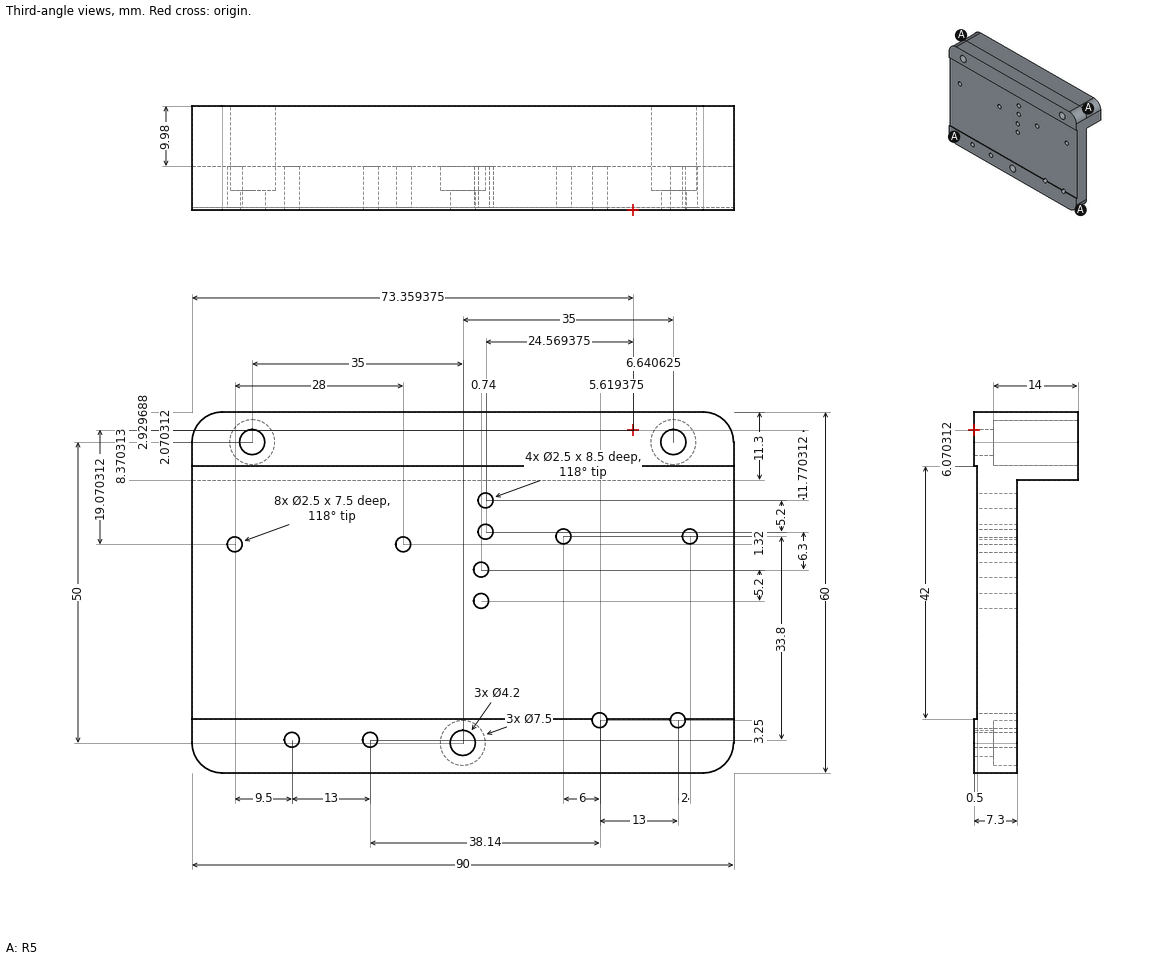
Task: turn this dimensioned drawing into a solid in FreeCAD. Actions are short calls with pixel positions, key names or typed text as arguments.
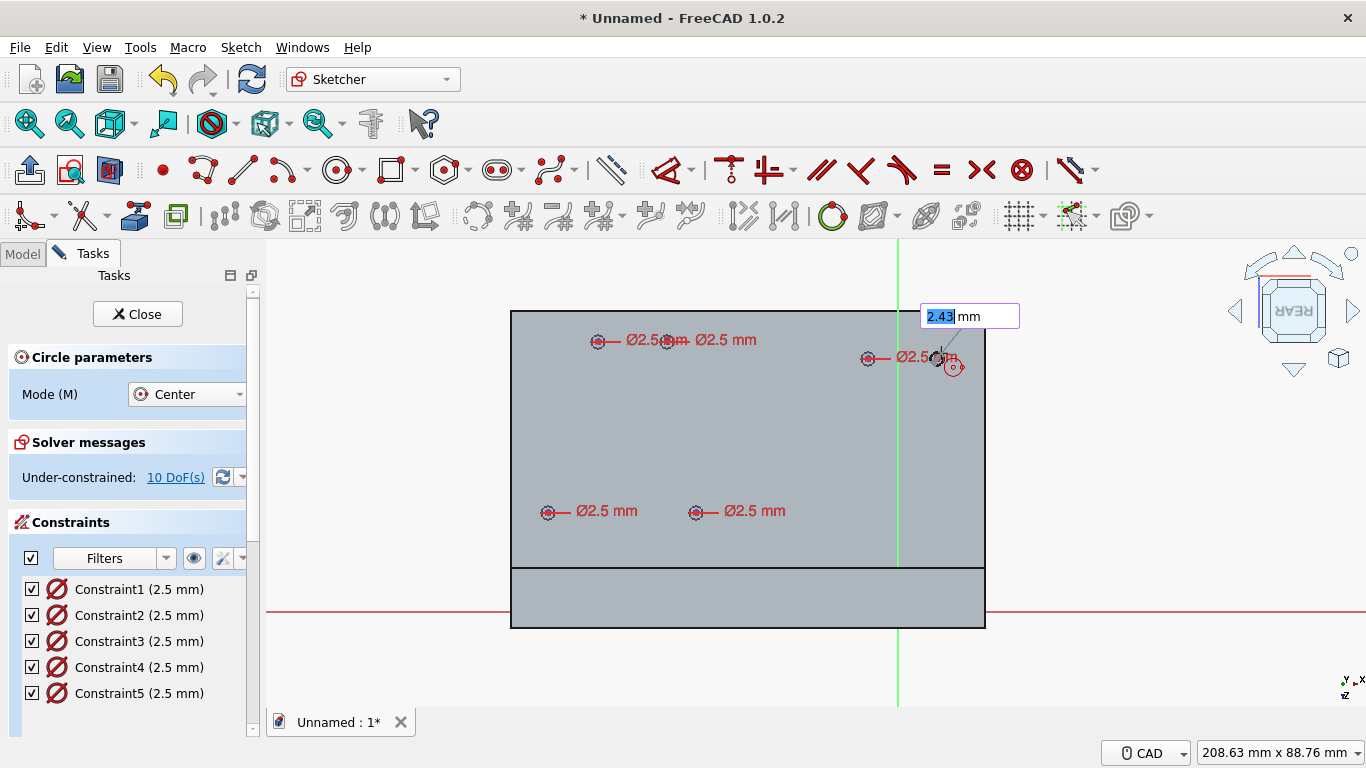
text(2.5)
key(Return)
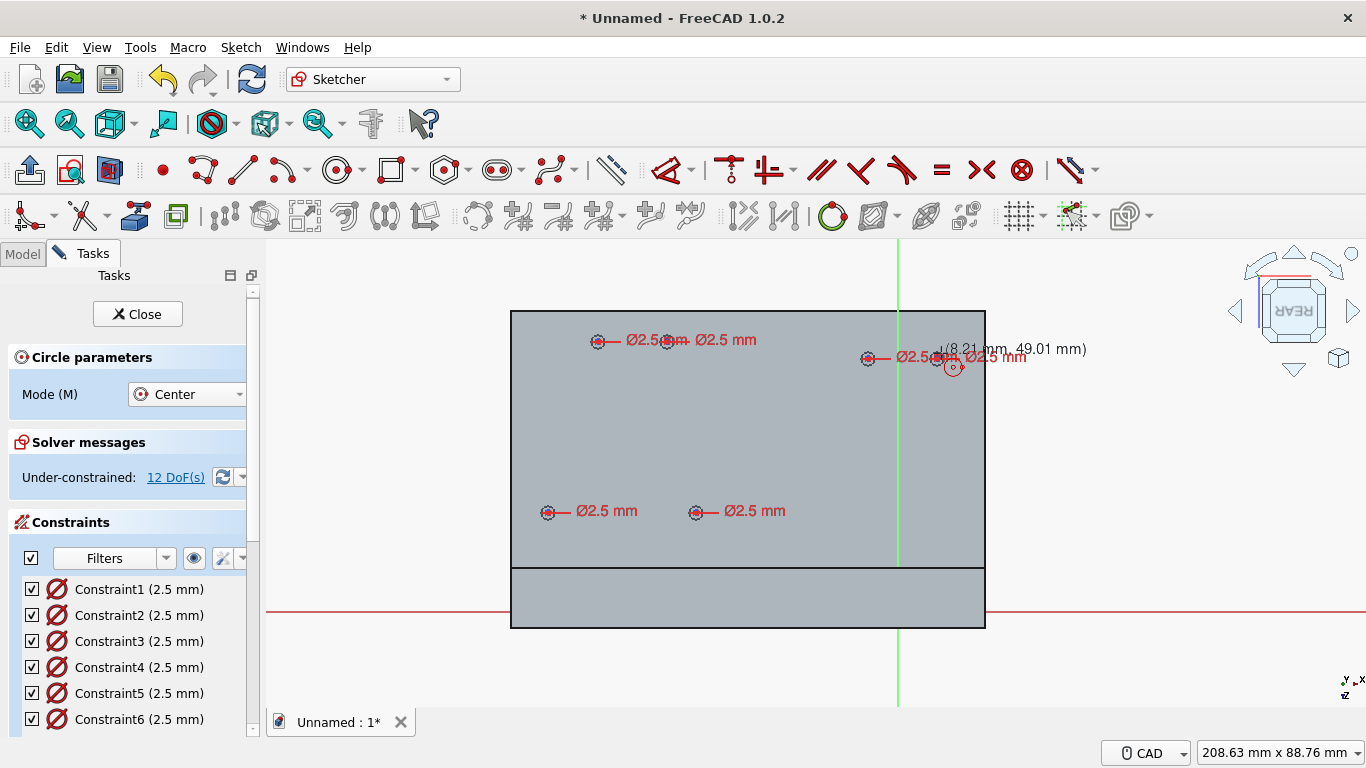
scroll(836, 519, up, 7)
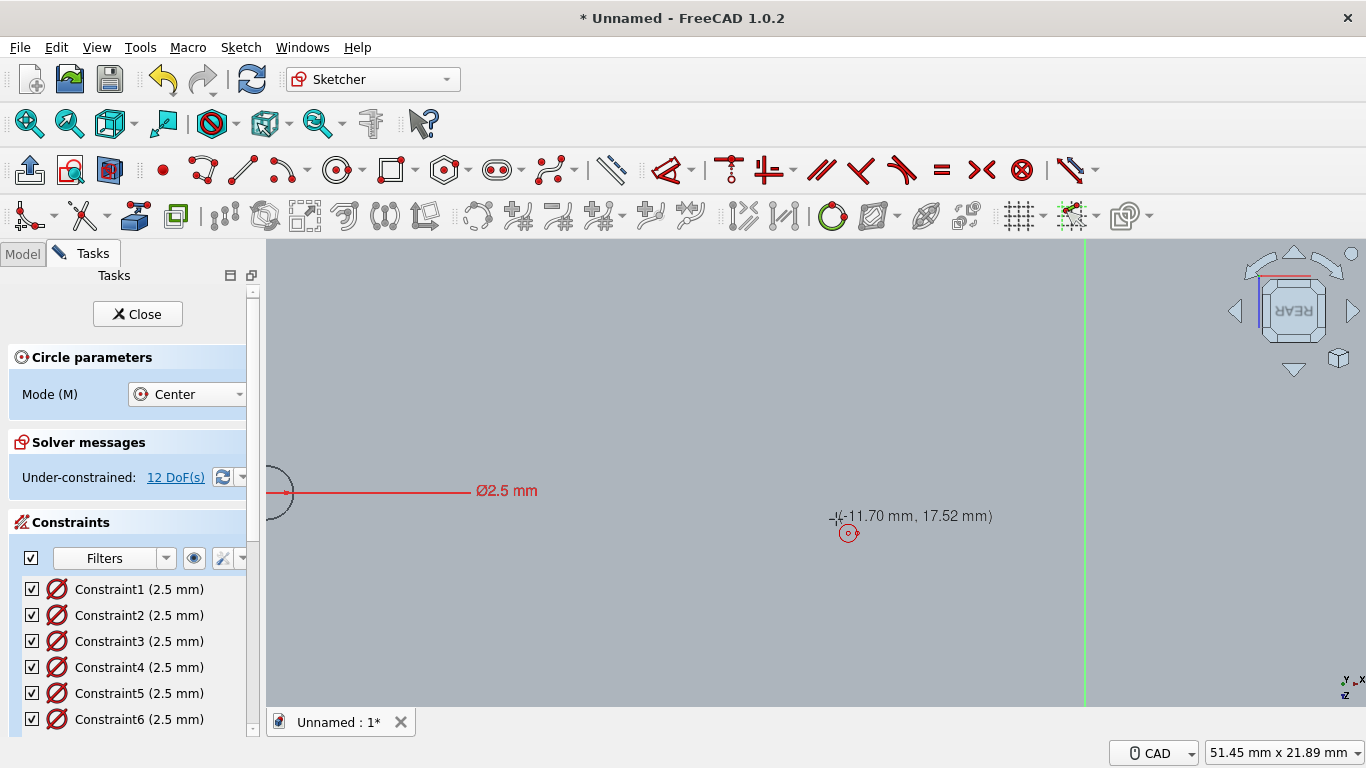
scroll(836, 519, down, 7)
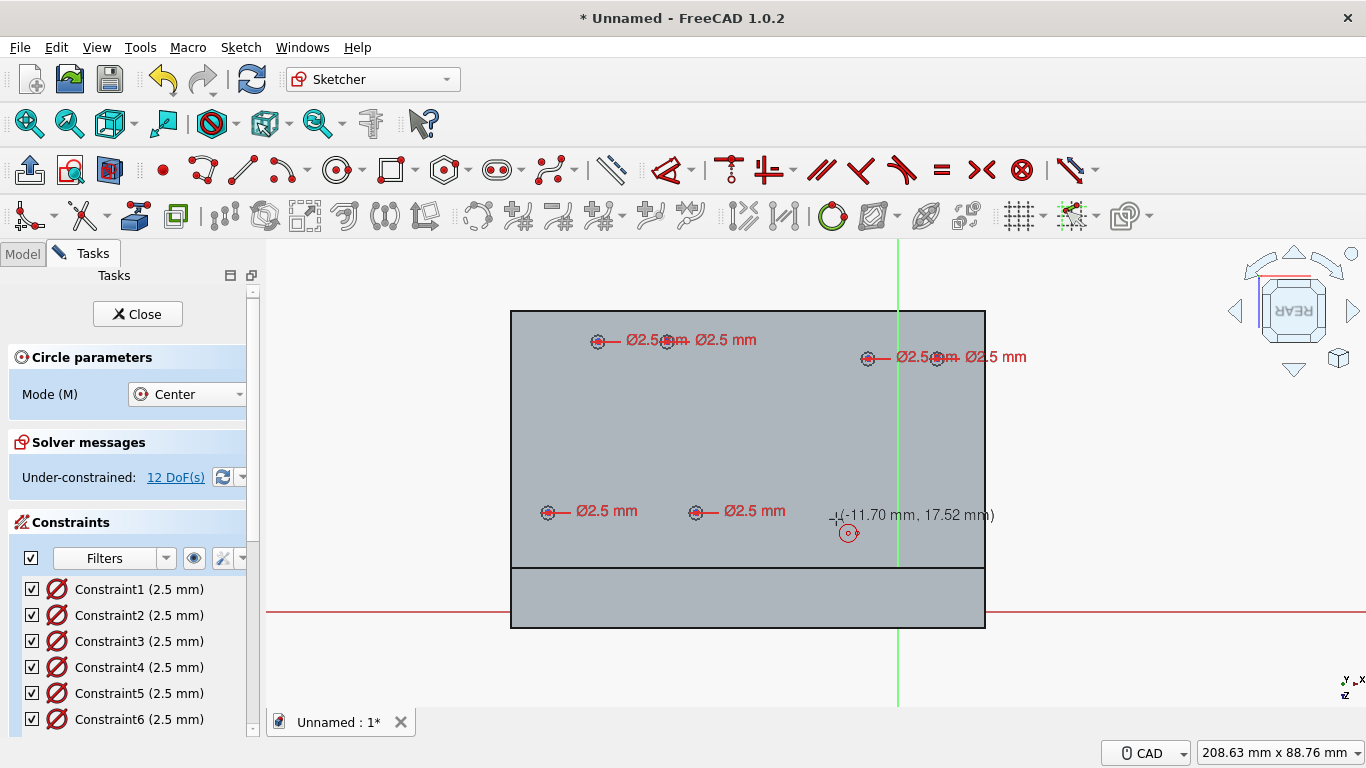
click(836, 519)
move(841, 514)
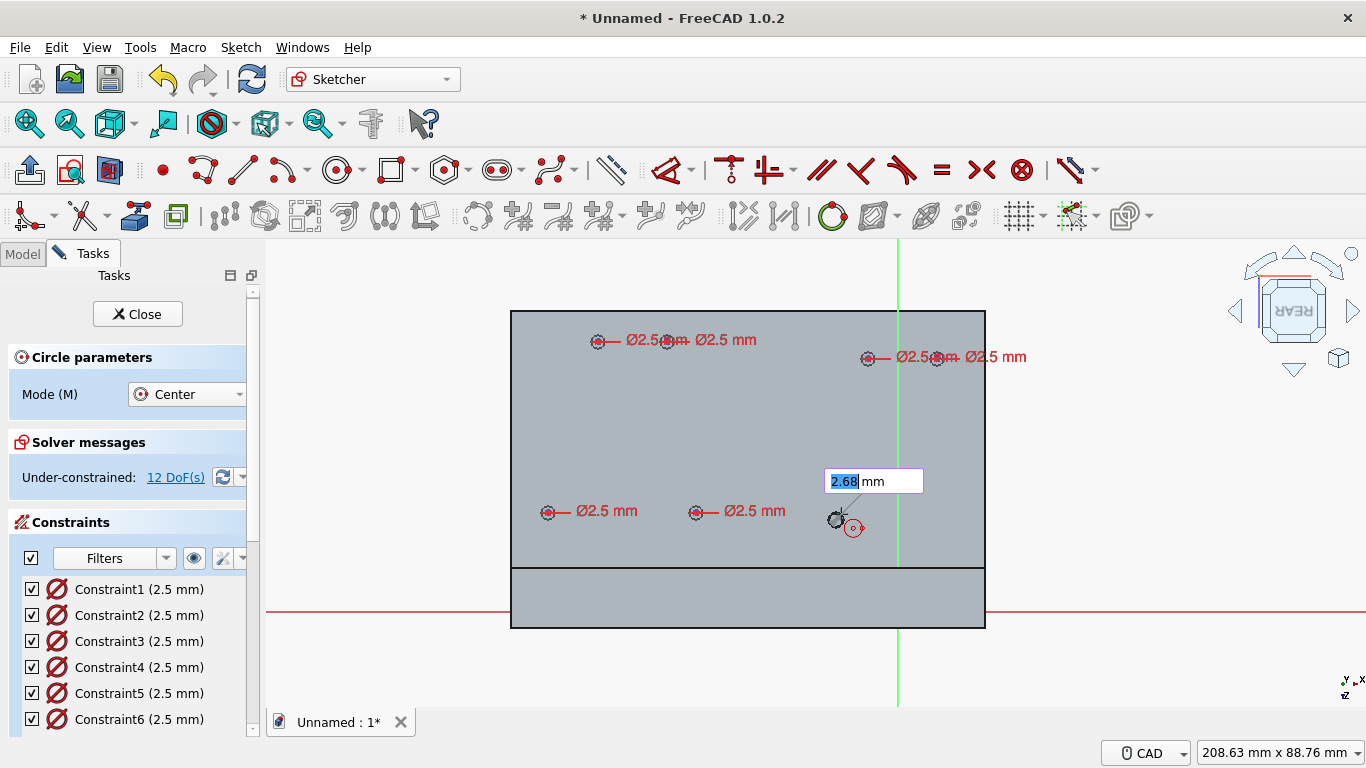
text(2.5)
key(Return)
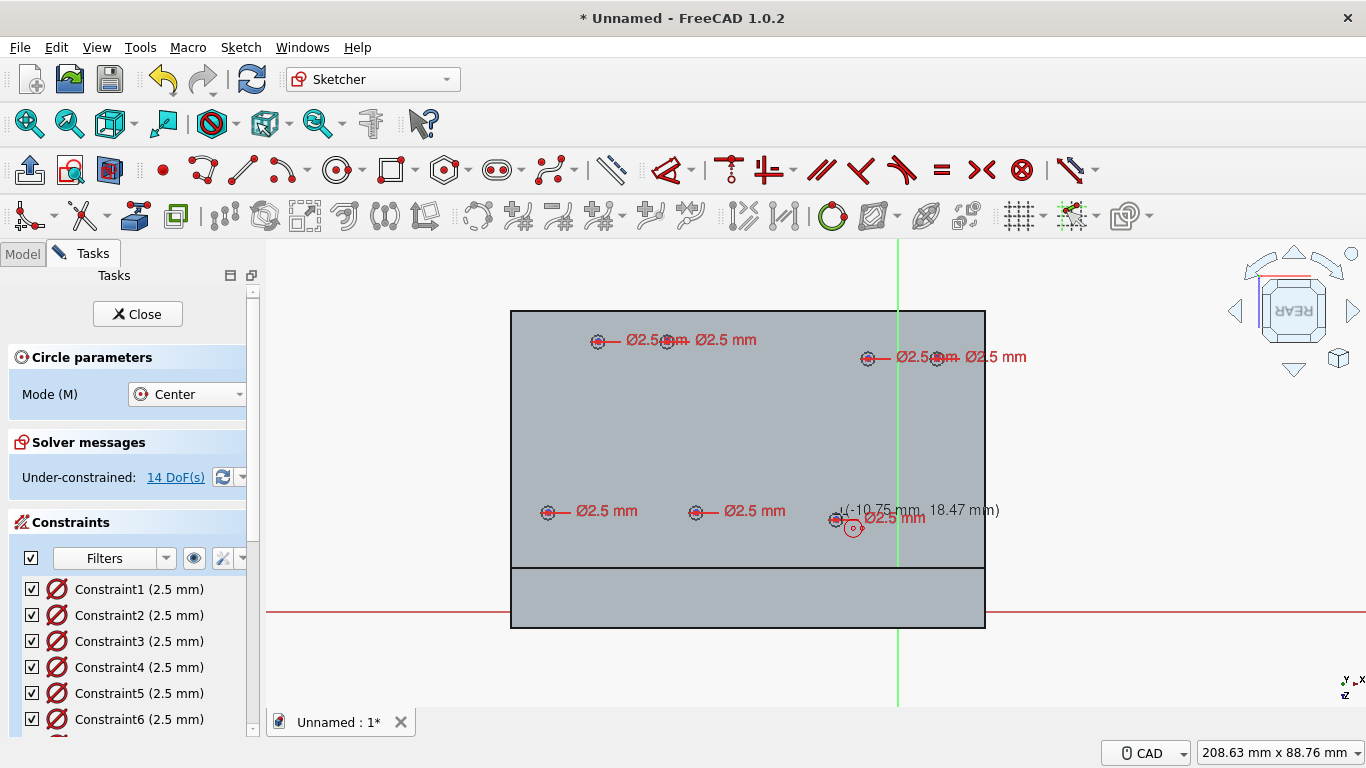
scroll(947, 519, up, 7)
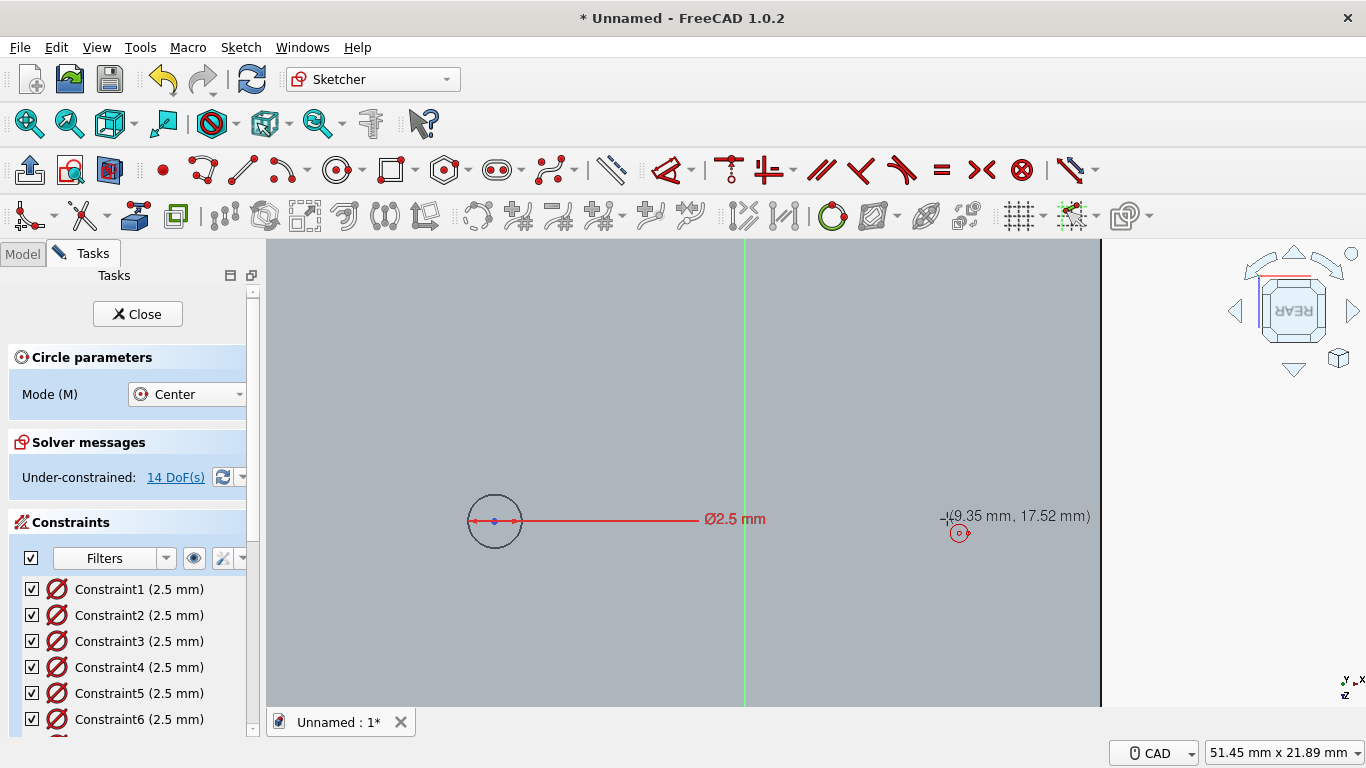
scroll(947, 519, down, 7)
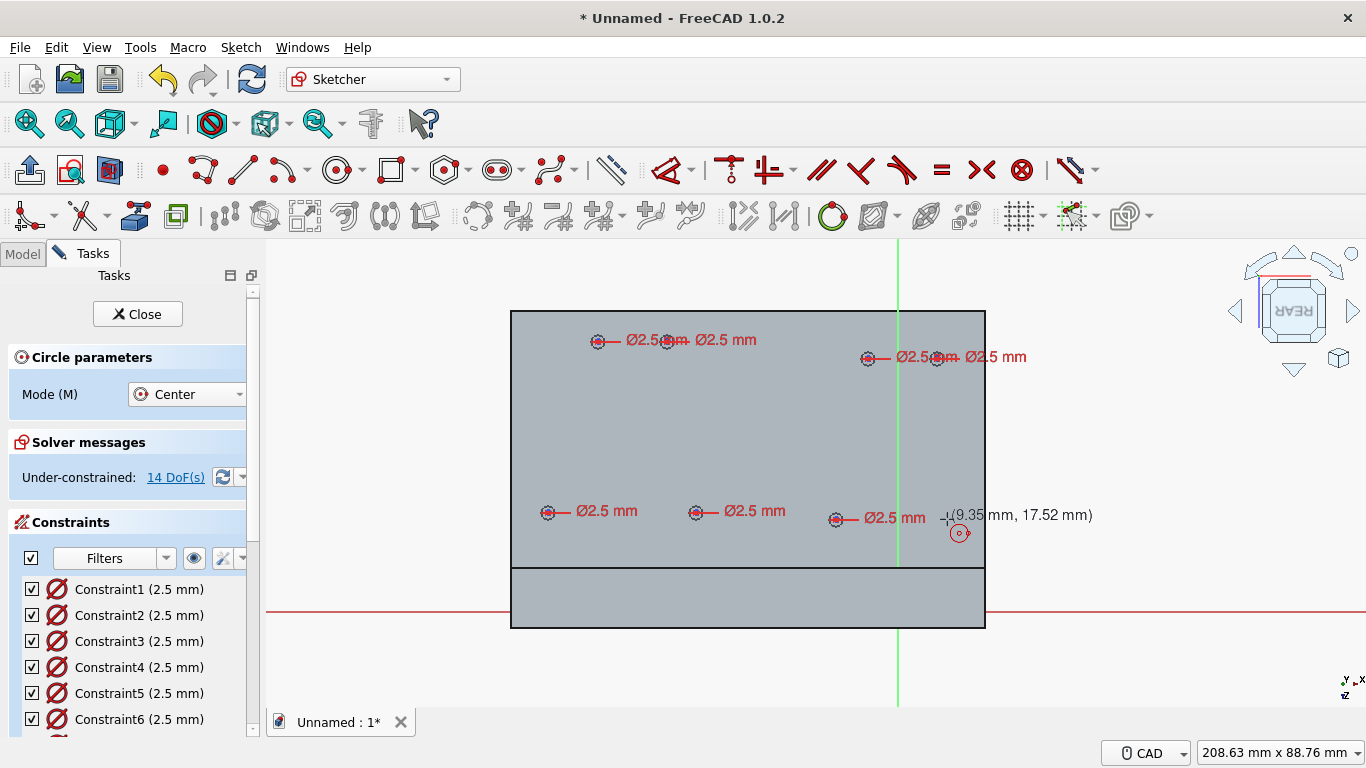
click(947, 519)
move(952, 514)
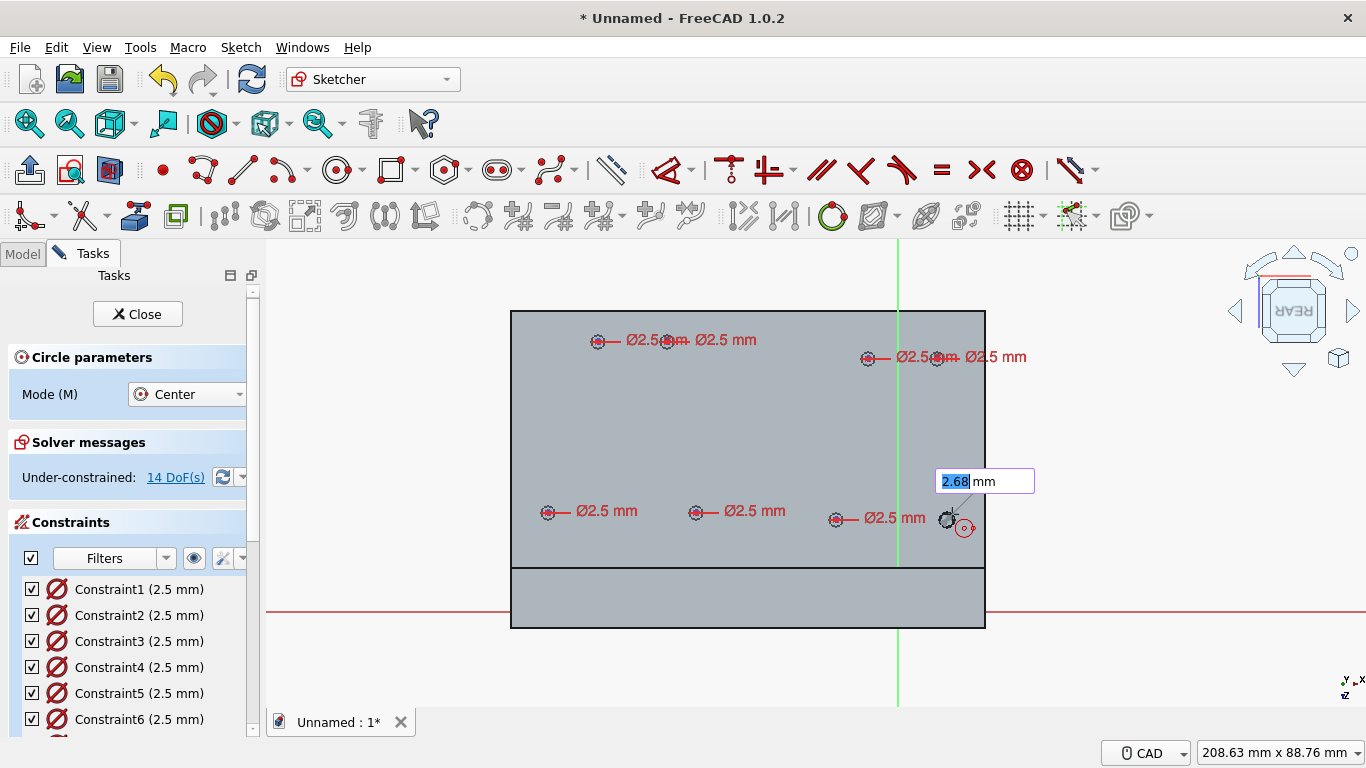
text(2.5)
key(Return)
key(Escape)